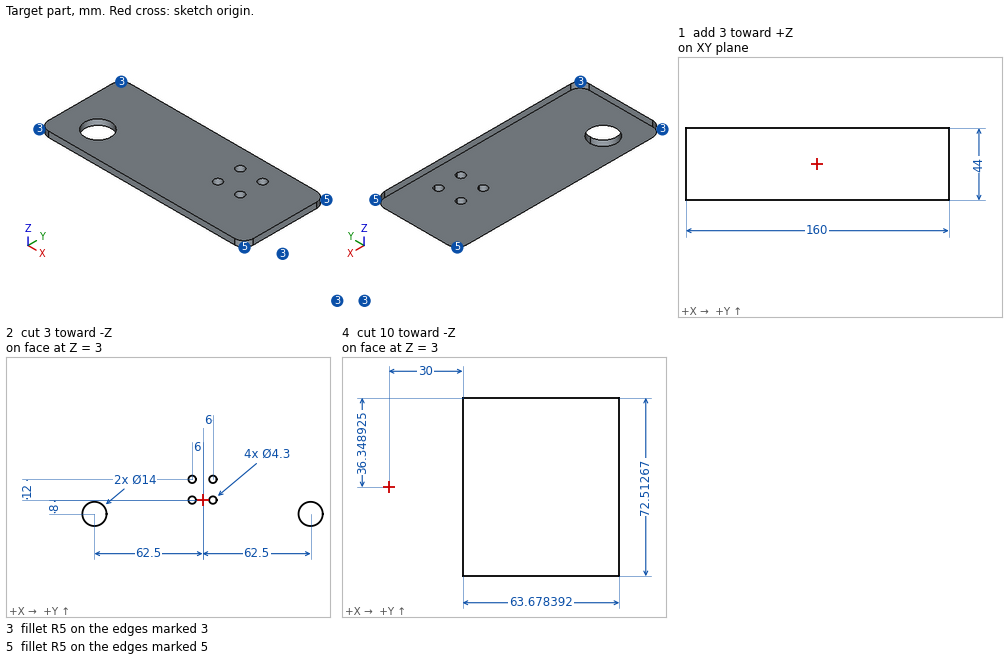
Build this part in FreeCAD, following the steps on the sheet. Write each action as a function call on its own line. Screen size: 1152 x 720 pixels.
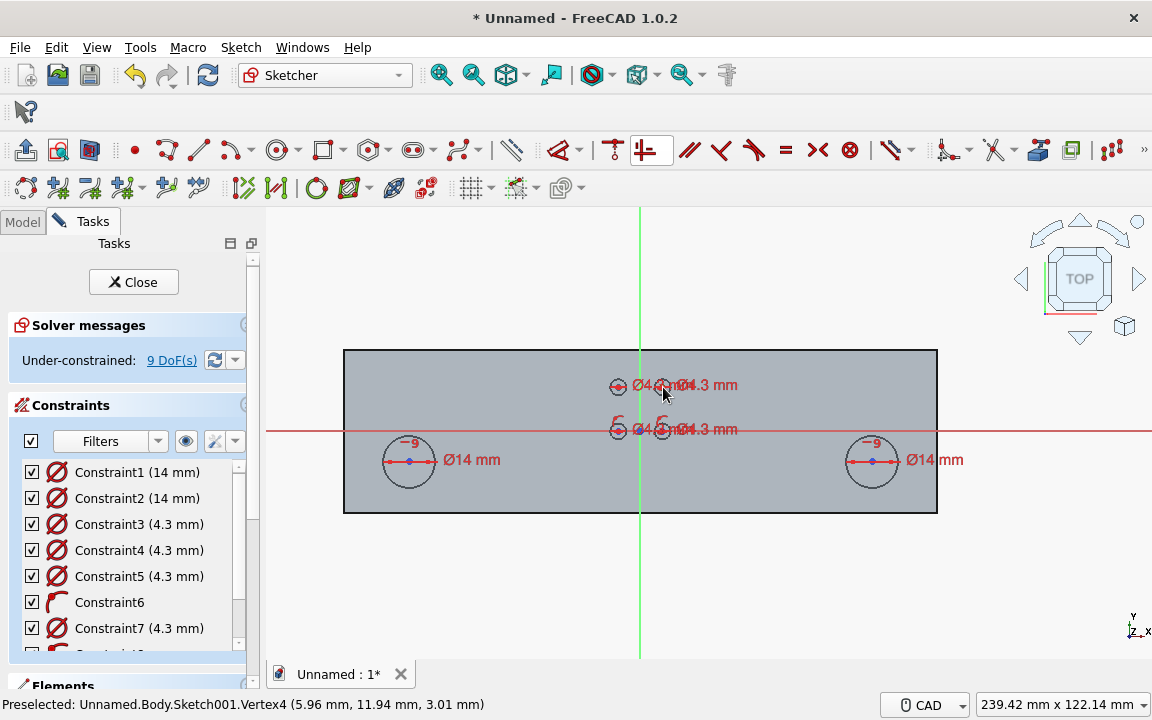
key(h)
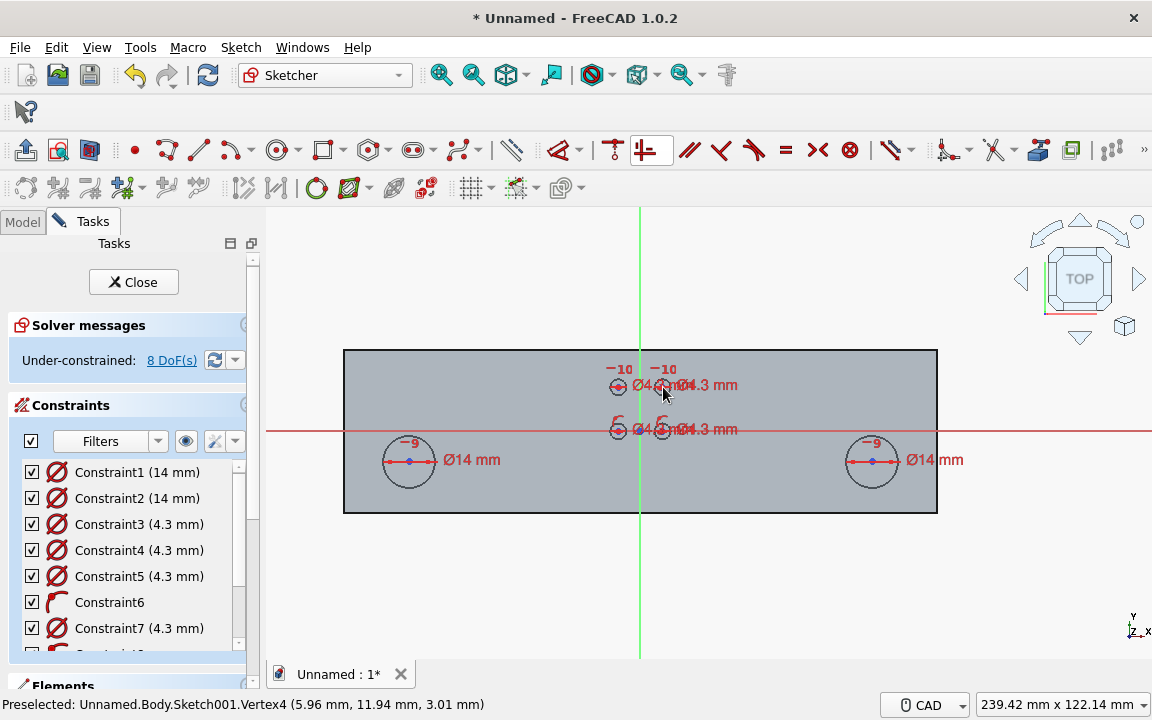
click(663, 387)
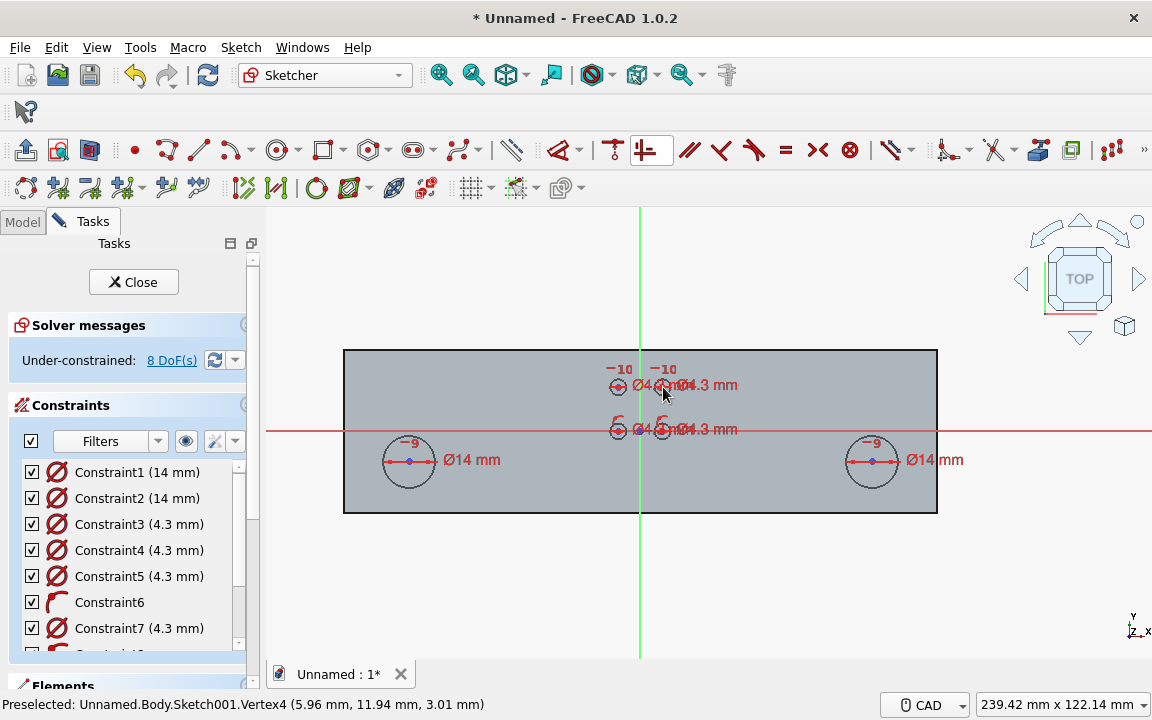
click(663, 431)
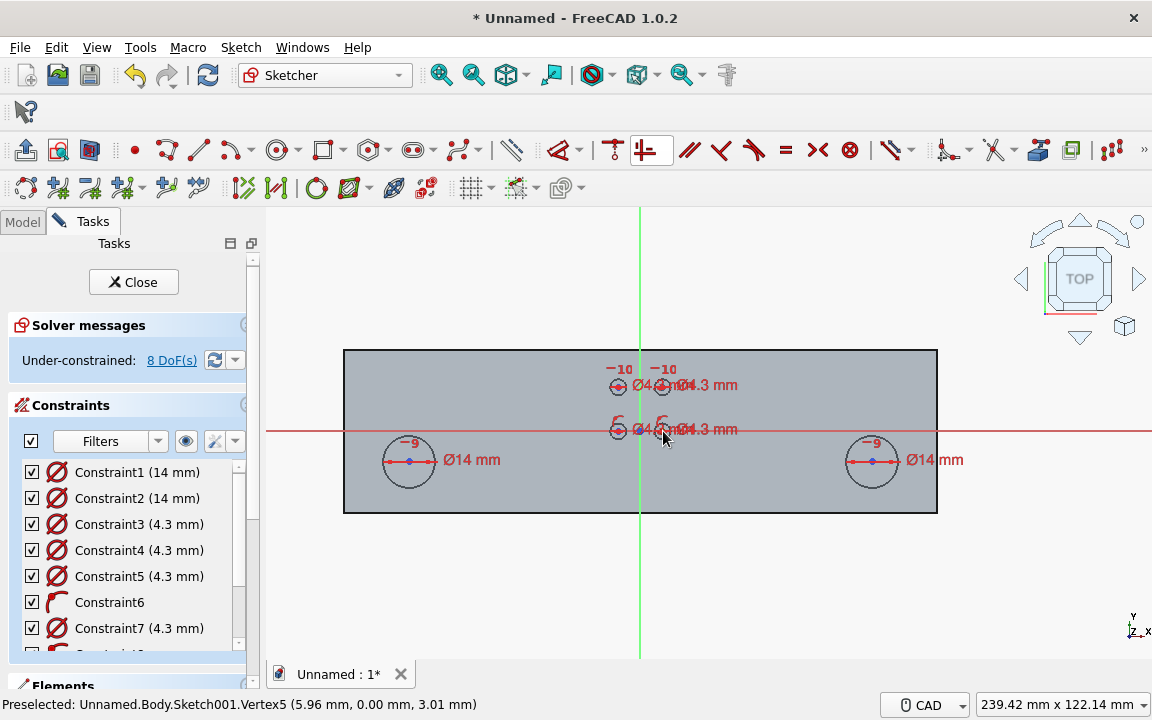
key(v)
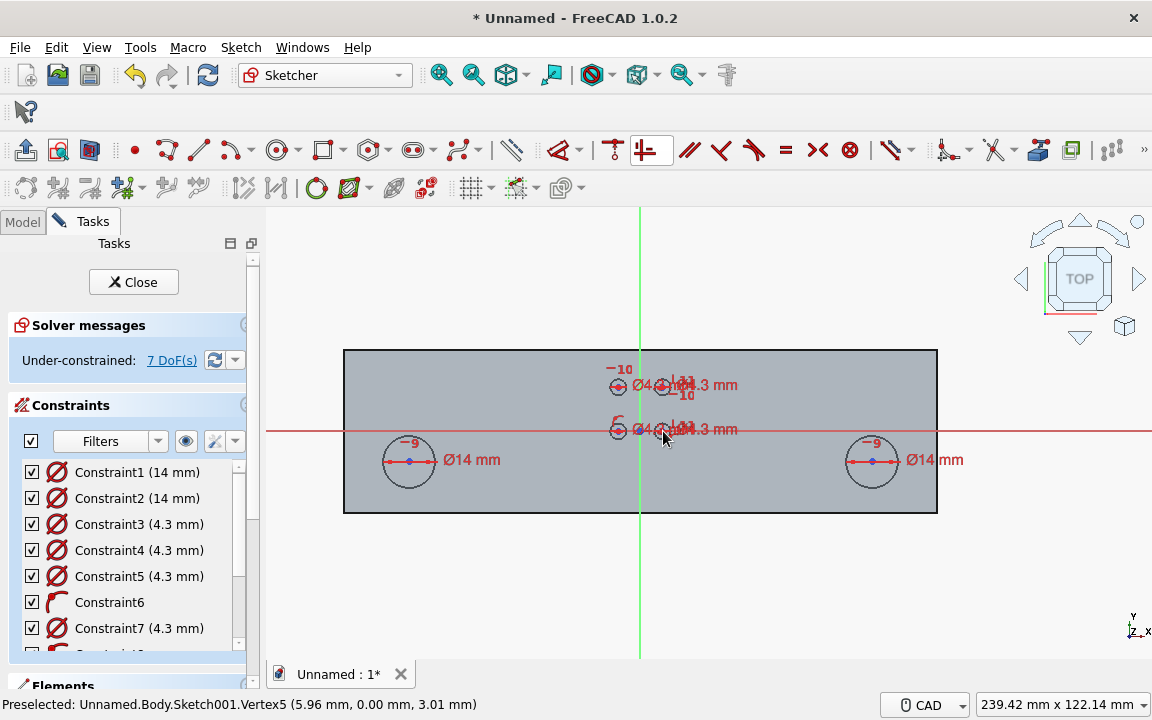
click(618, 387)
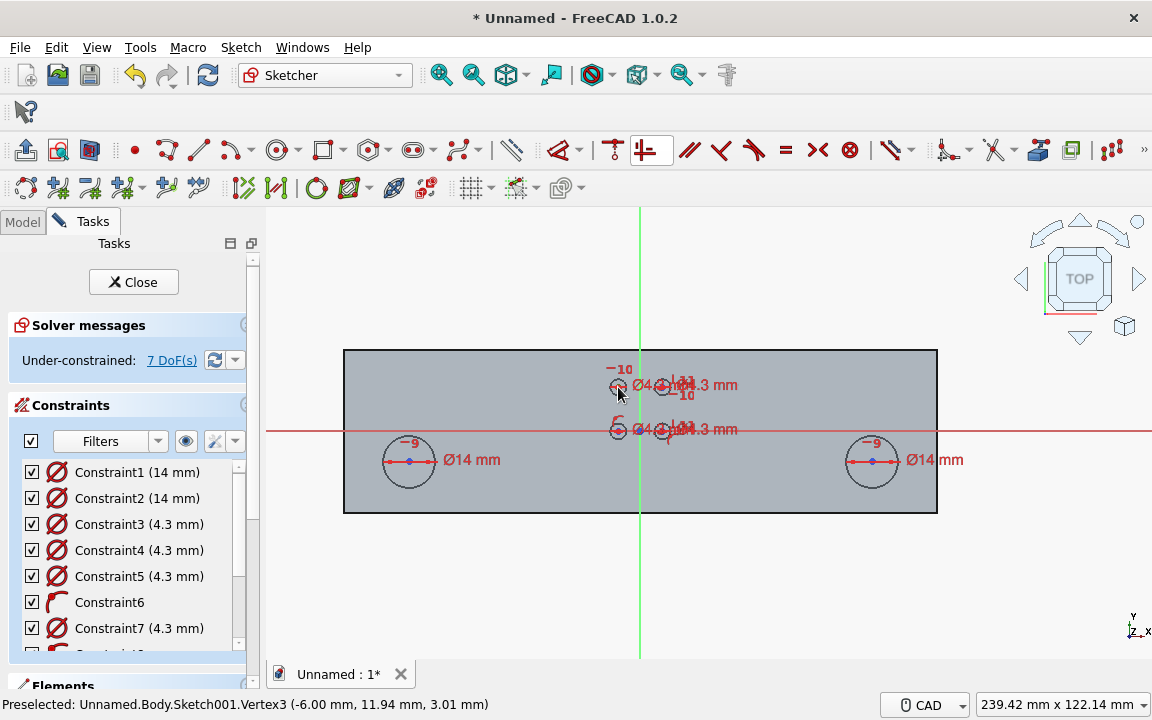
click(618, 431)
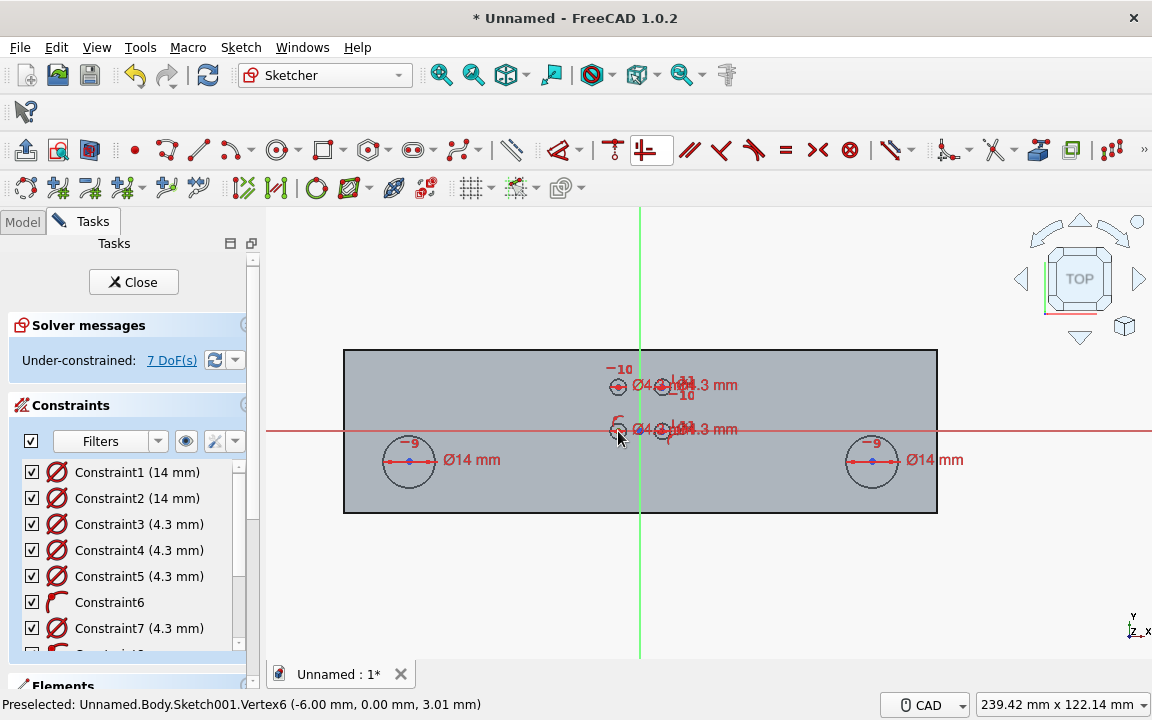
click(668, 150)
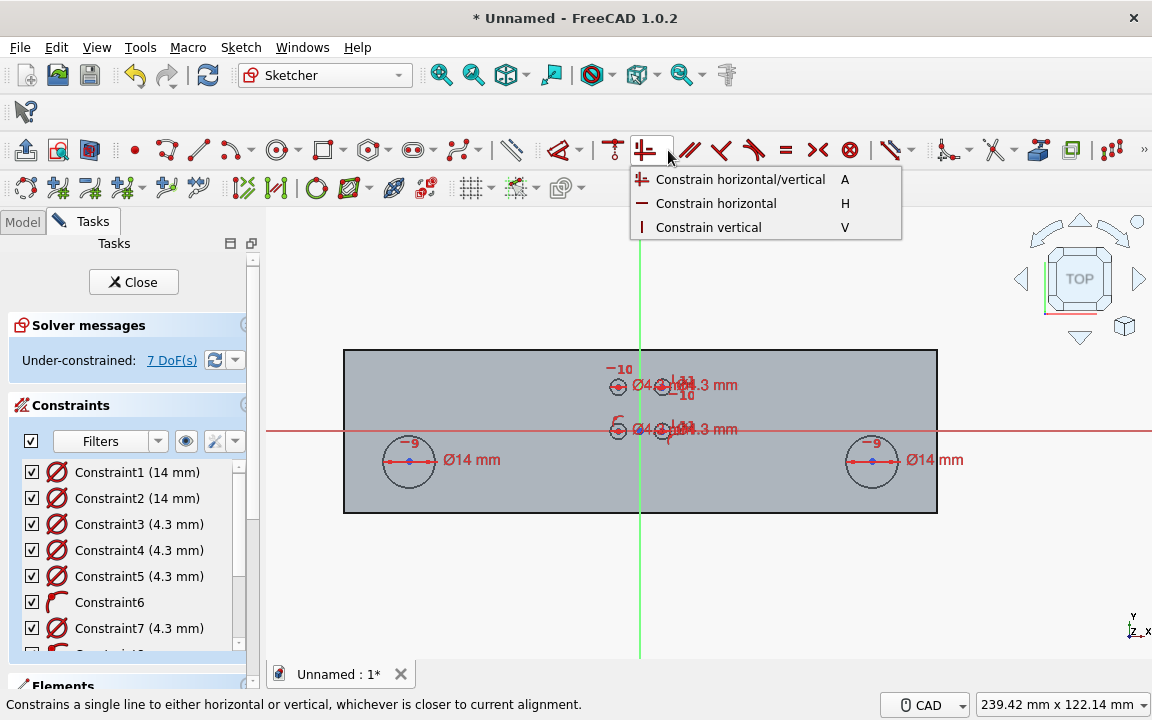
click(766, 227)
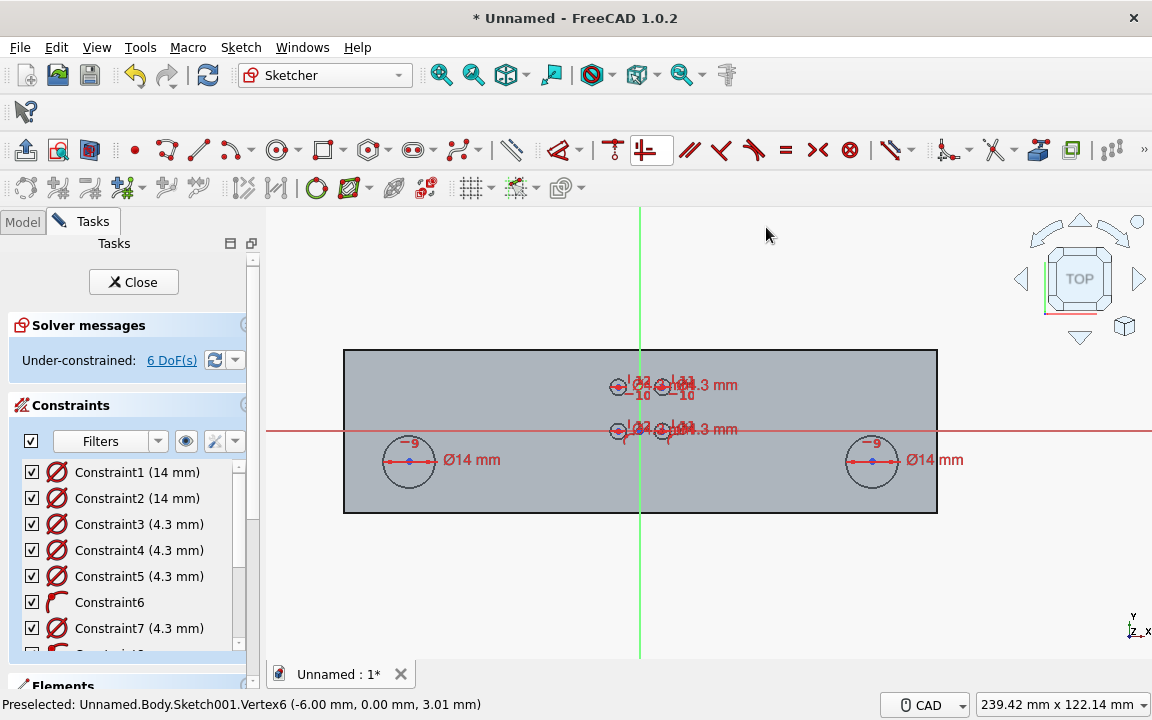
click(558, 150)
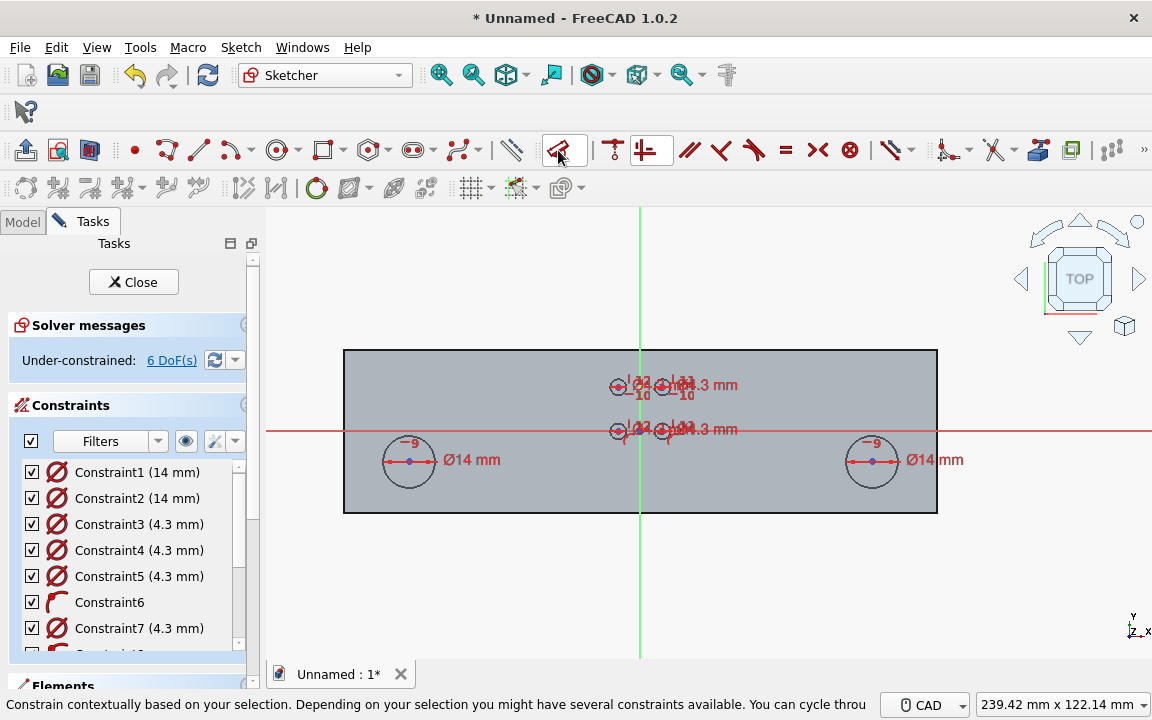
scroll(409, 462, up, 2)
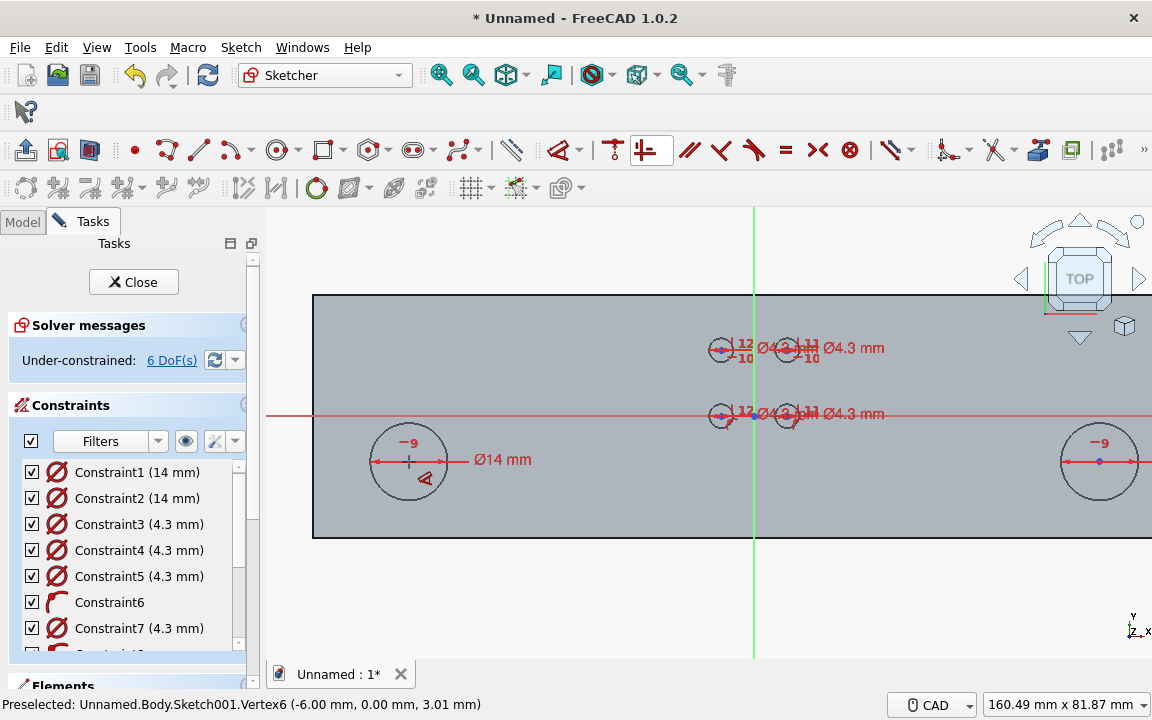
click(409, 462)
click(788, 449)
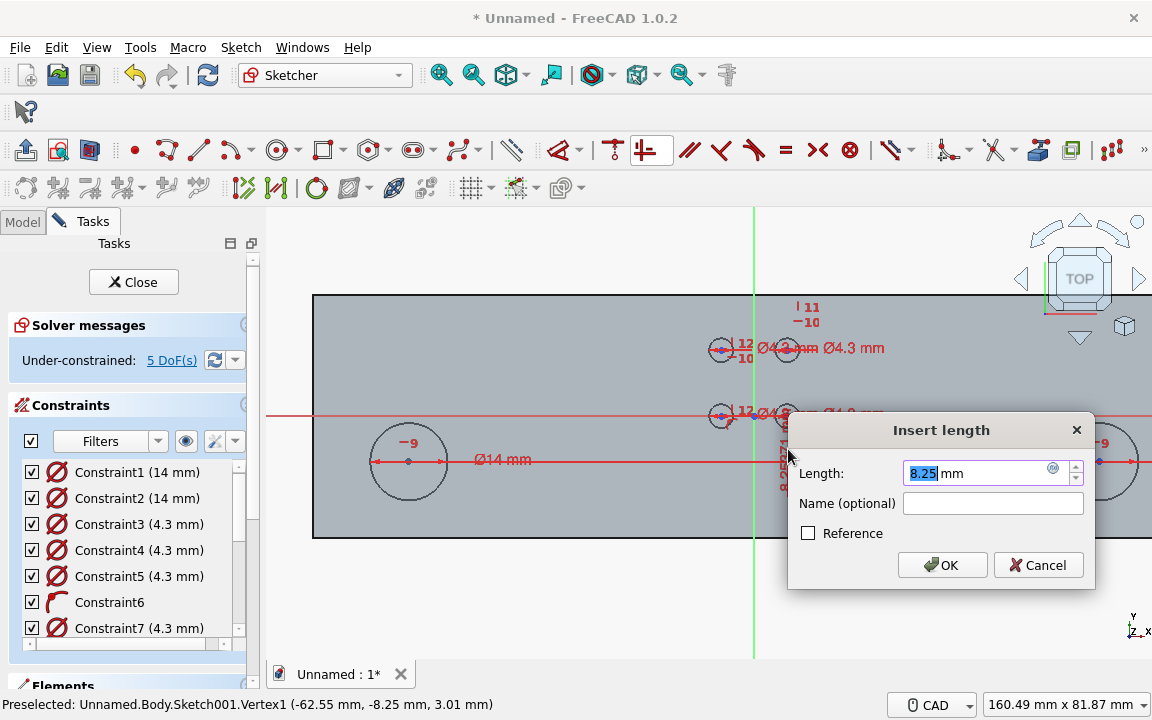
text(8)
key(Return)